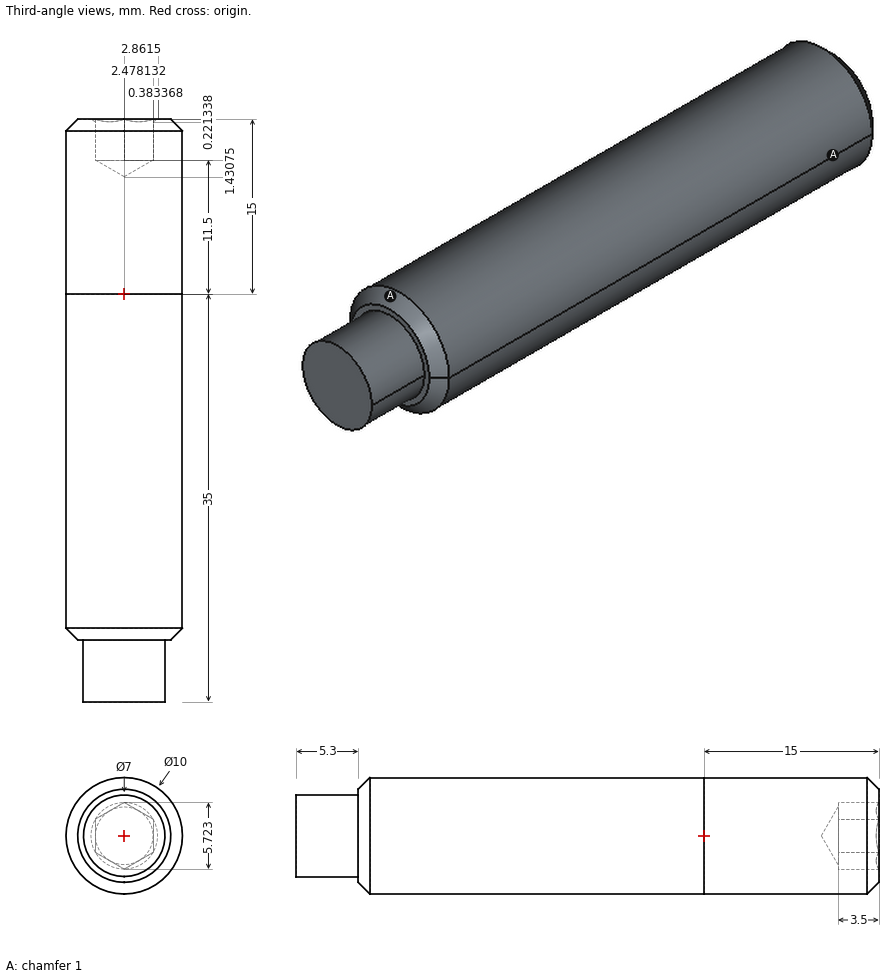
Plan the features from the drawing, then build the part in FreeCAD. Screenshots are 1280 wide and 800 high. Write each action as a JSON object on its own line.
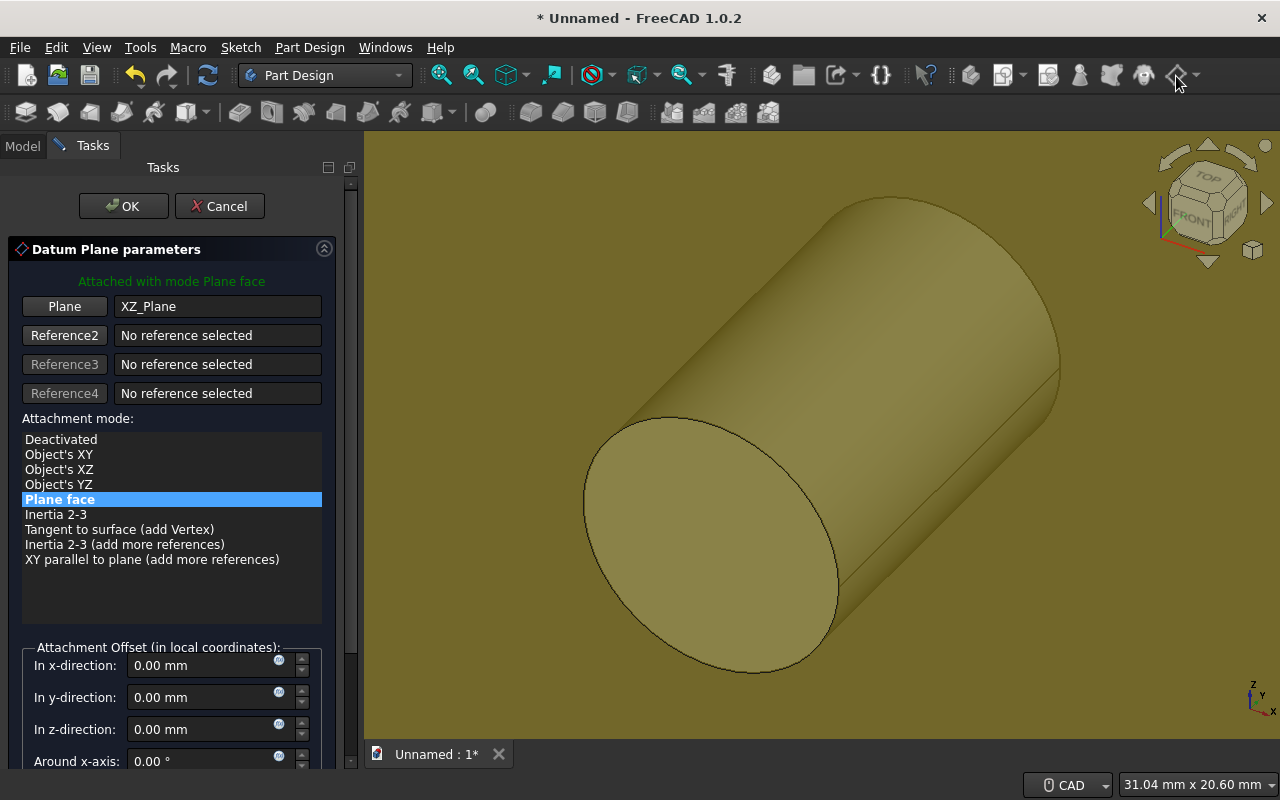
{"action": "triple_click", "coordinate": [210, 729]}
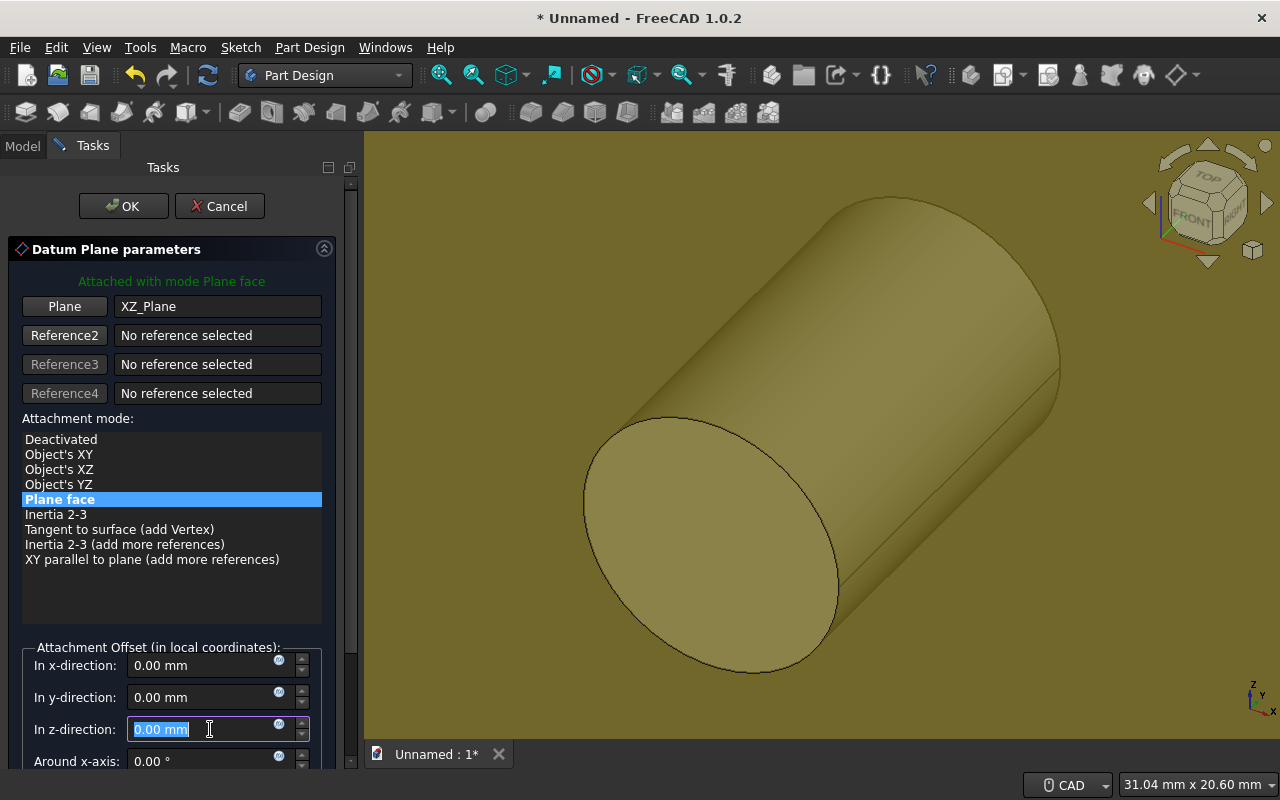
{"action": "type", "text": "35"}
{"action": "key", "text": "Tab"}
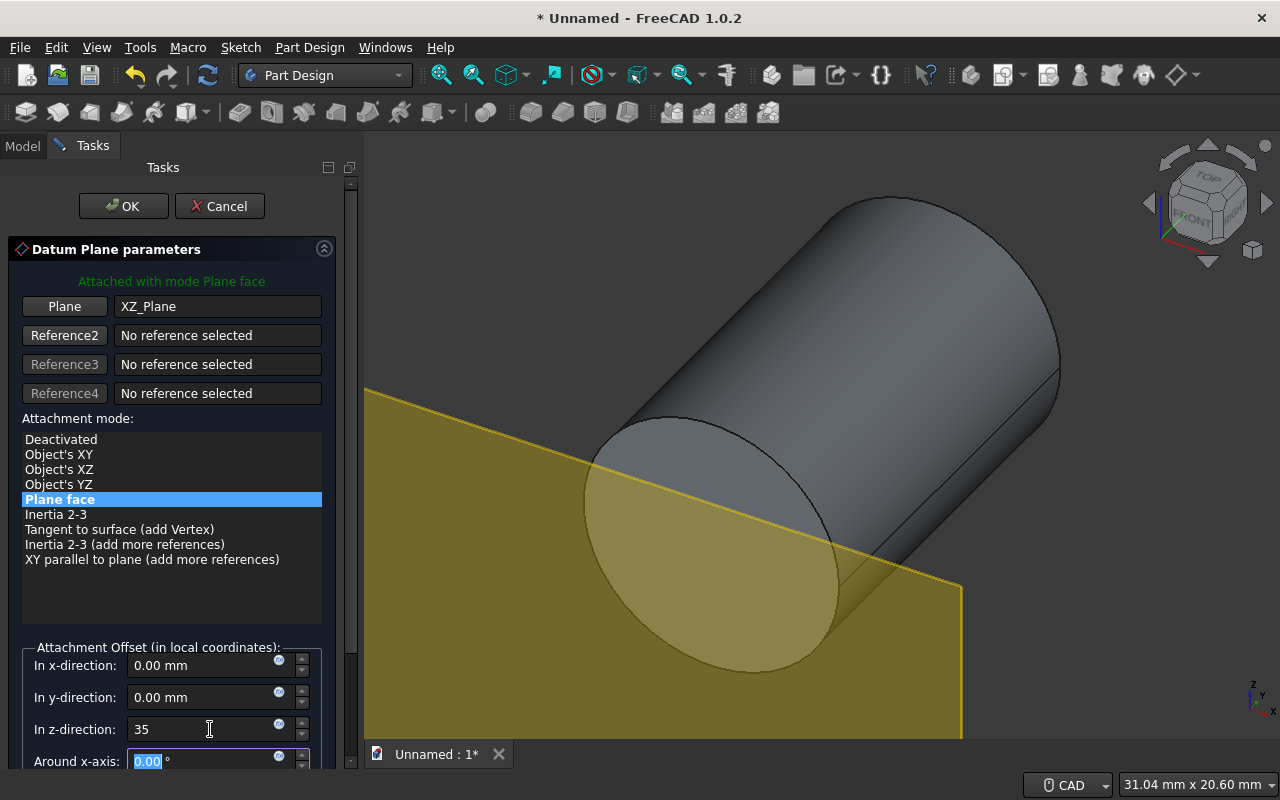
{"action": "left_click", "coordinate": [124, 206]}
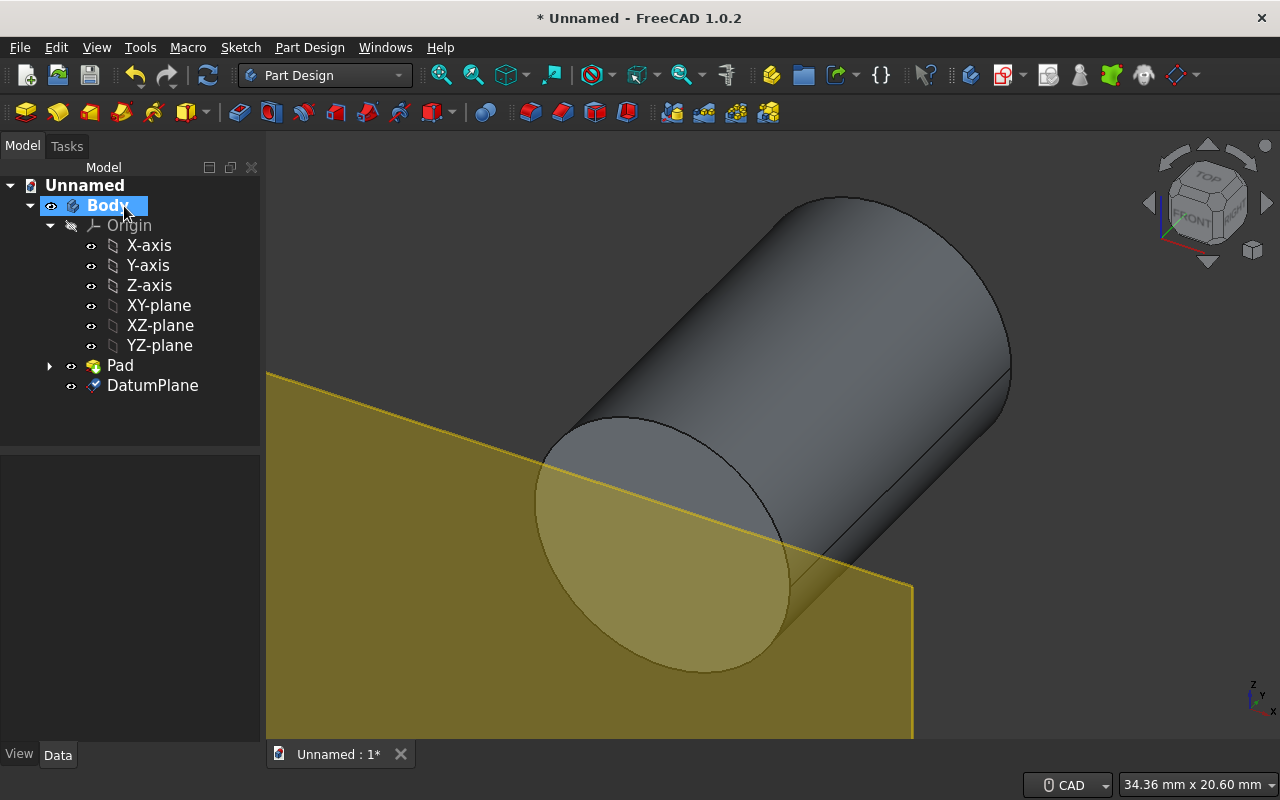
{"action": "left_click", "coordinate": [116, 386]}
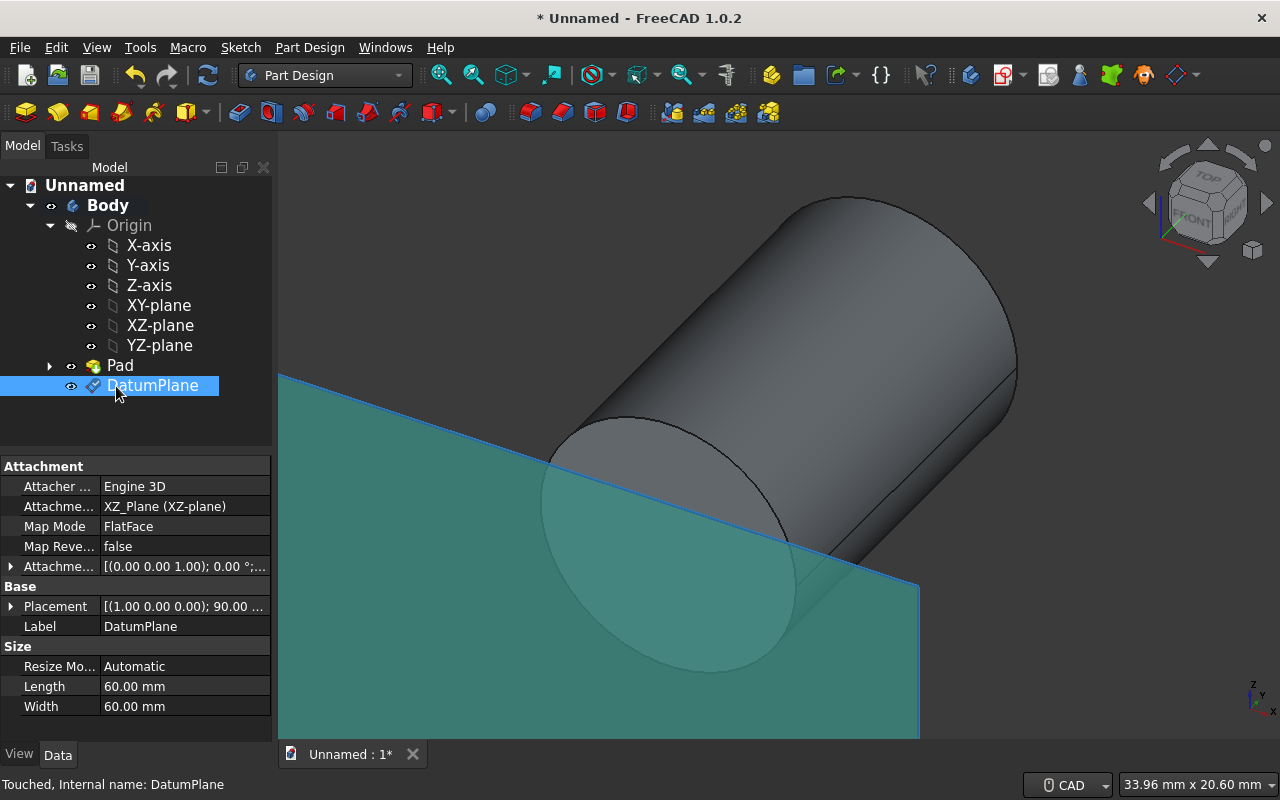
{"action": "left_click", "coordinate": [1004, 76]}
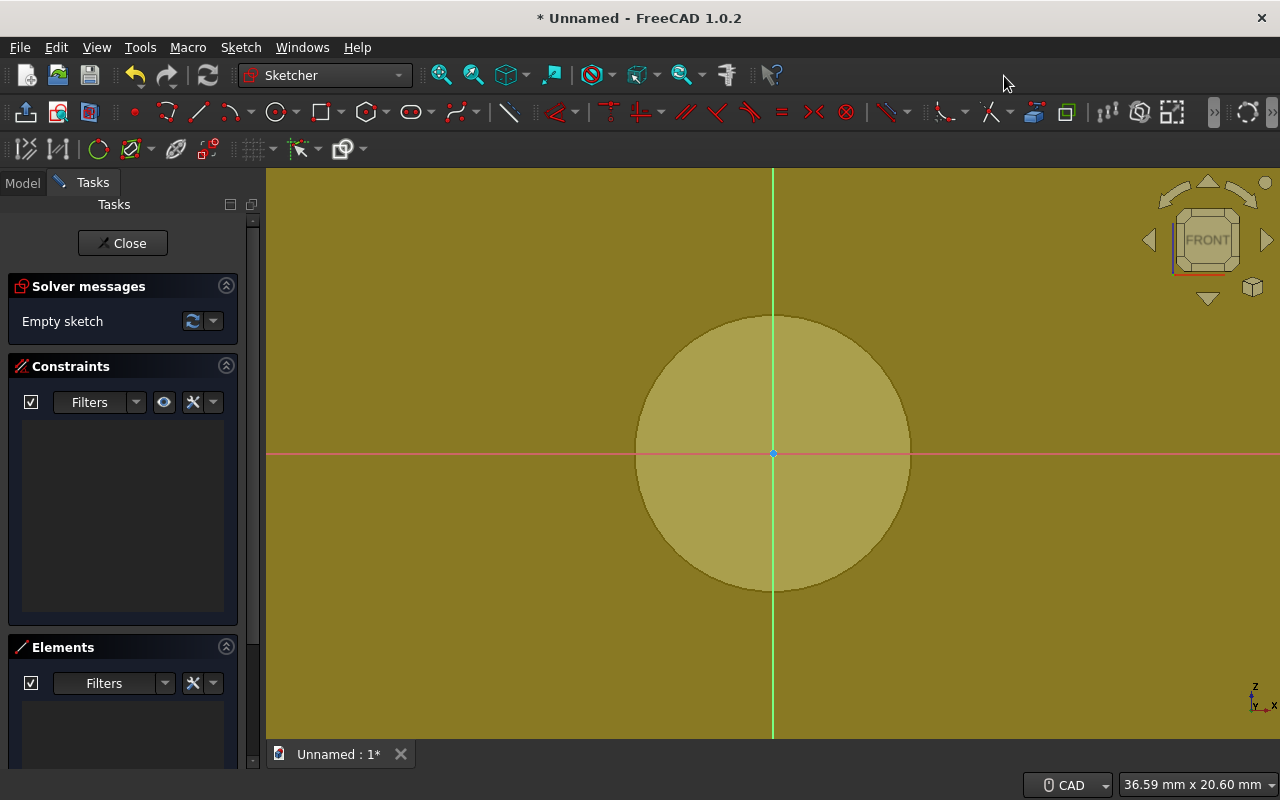
{"action": "left_click", "coordinate": [276, 112]}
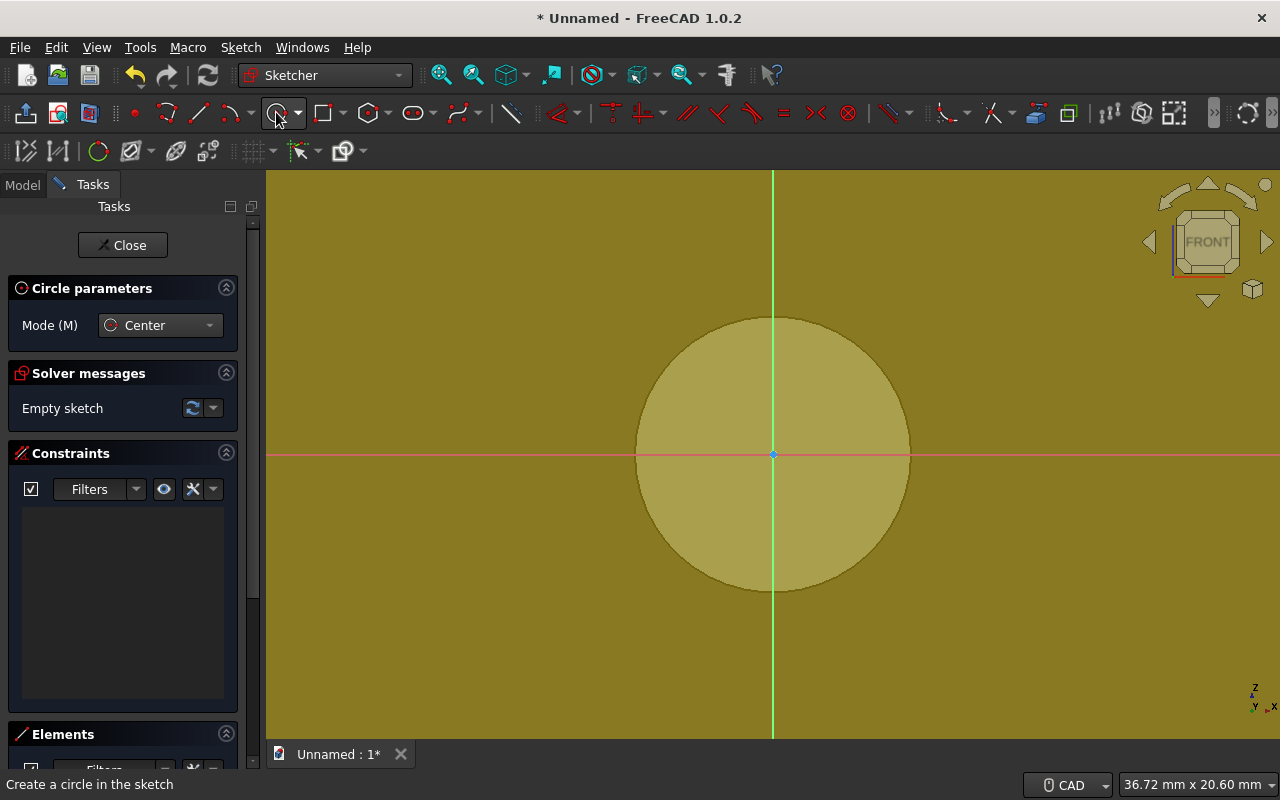
{"action": "left_click", "coordinate": [773, 455]}
{"action": "left_click", "coordinate": [871, 357]}
{"action": "key", "text": "Escape"}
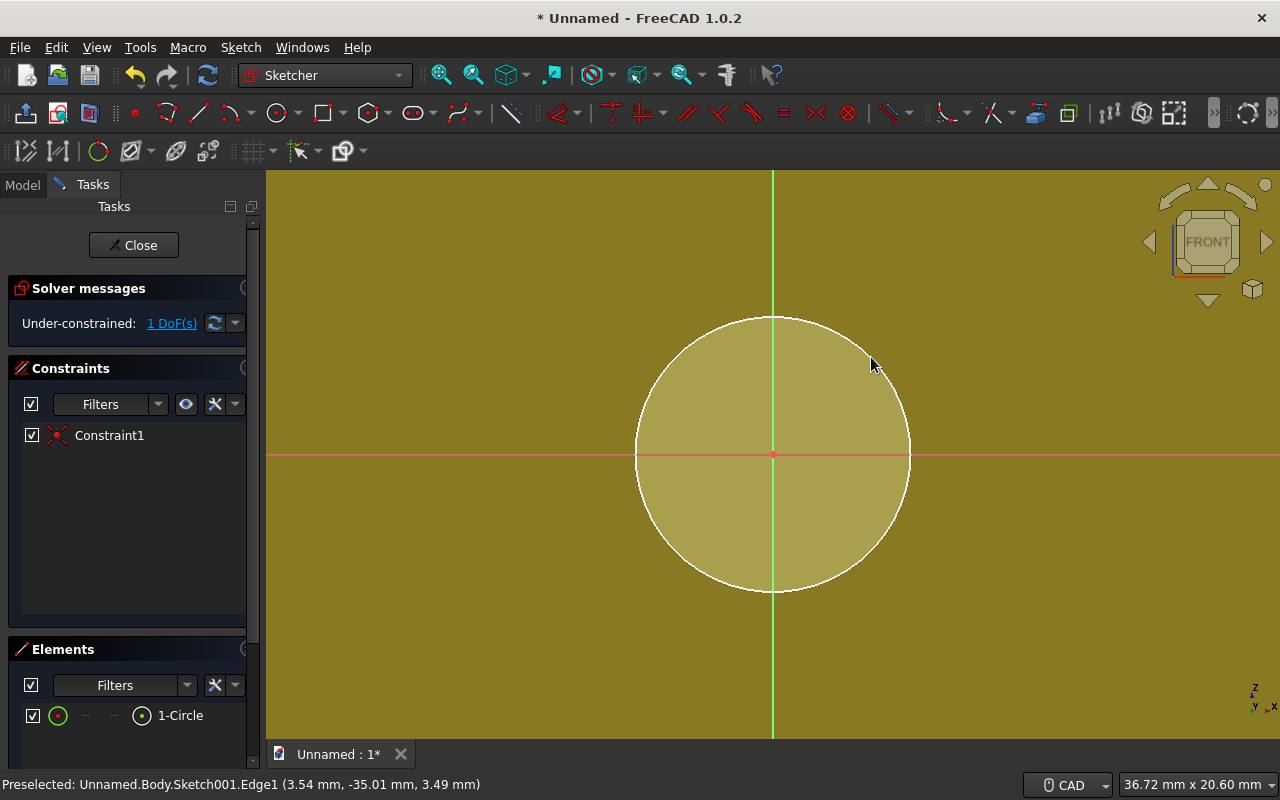
{"action": "left_click", "coordinate": [870, 357]}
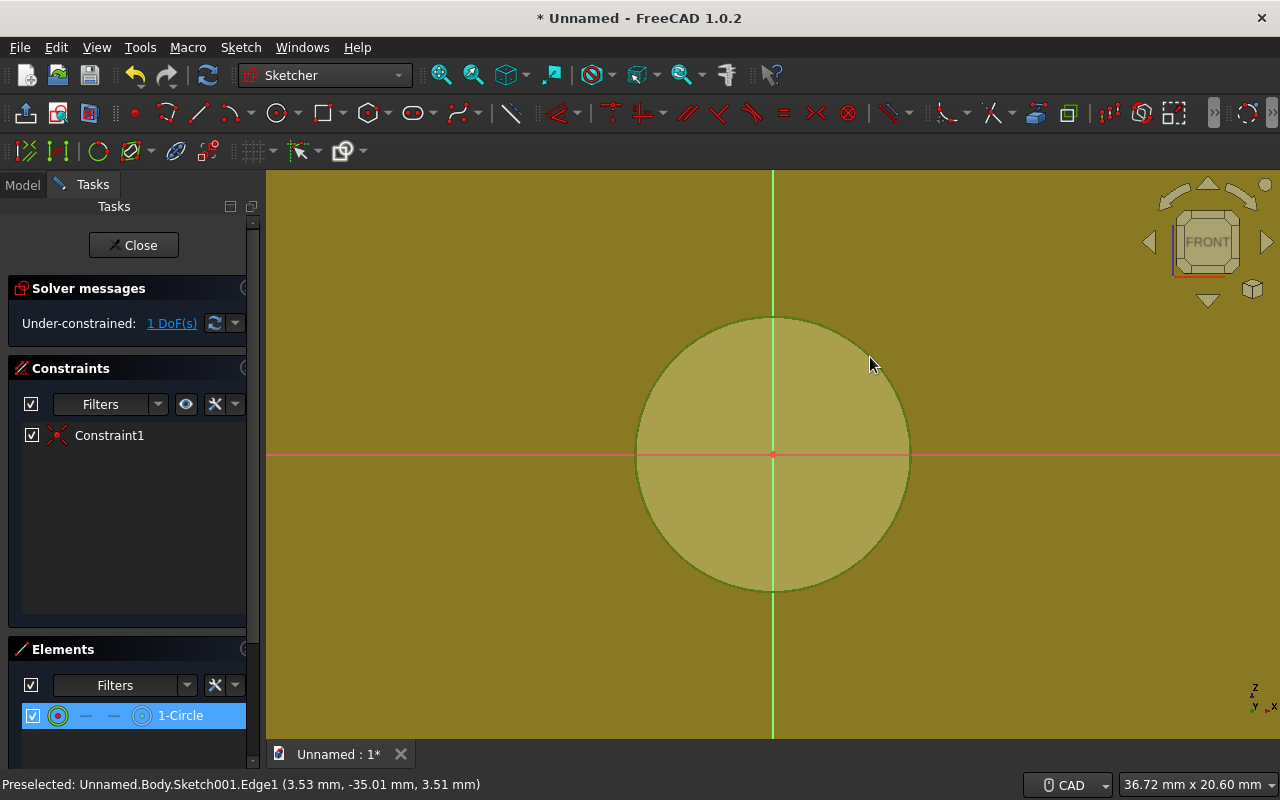
{"action": "left_click", "coordinate": [580, 114]}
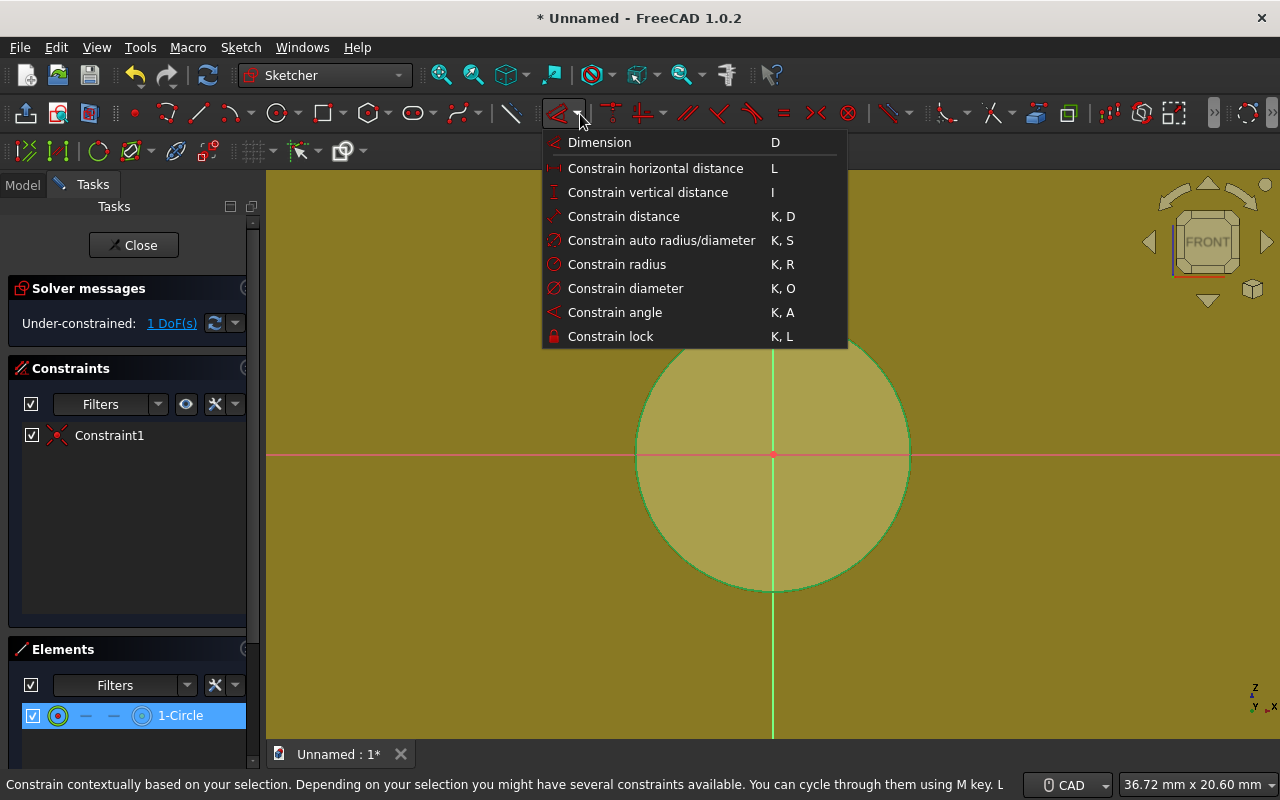
{"action": "left_click", "coordinate": [695, 288]}